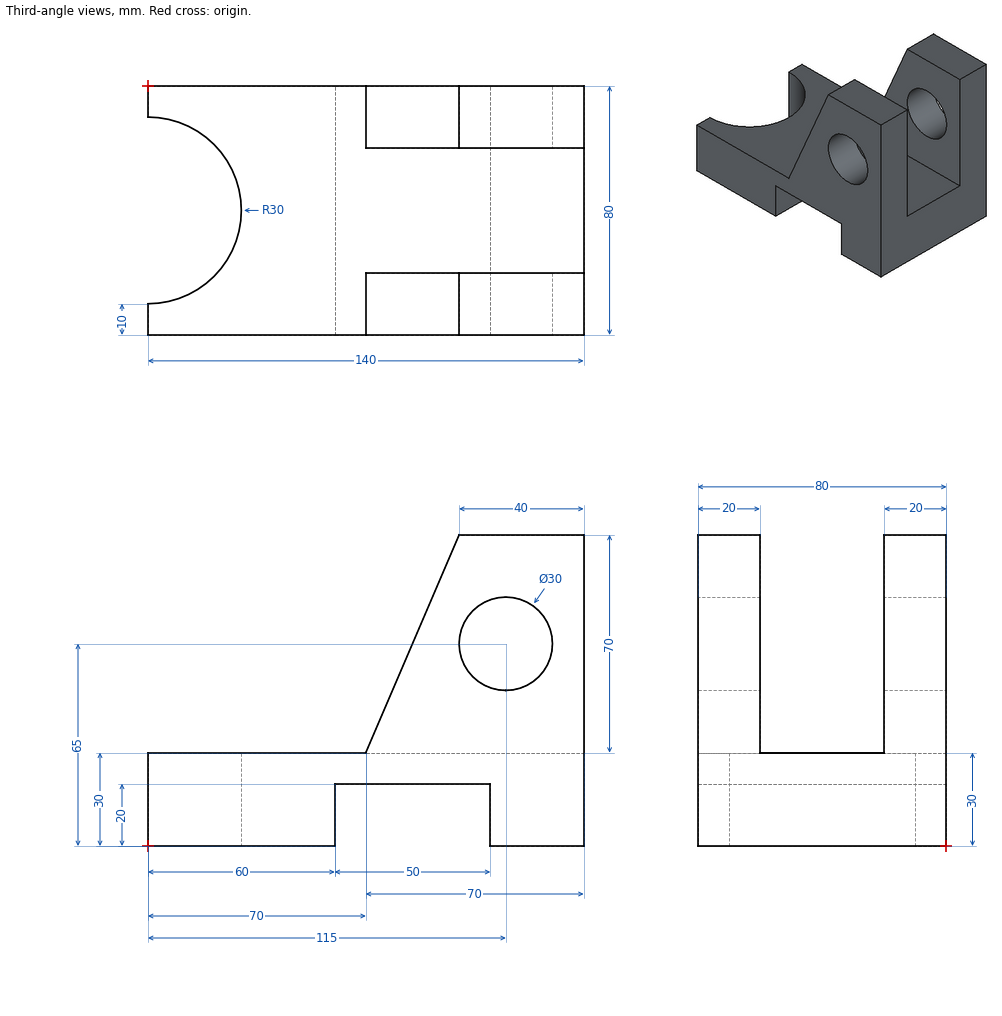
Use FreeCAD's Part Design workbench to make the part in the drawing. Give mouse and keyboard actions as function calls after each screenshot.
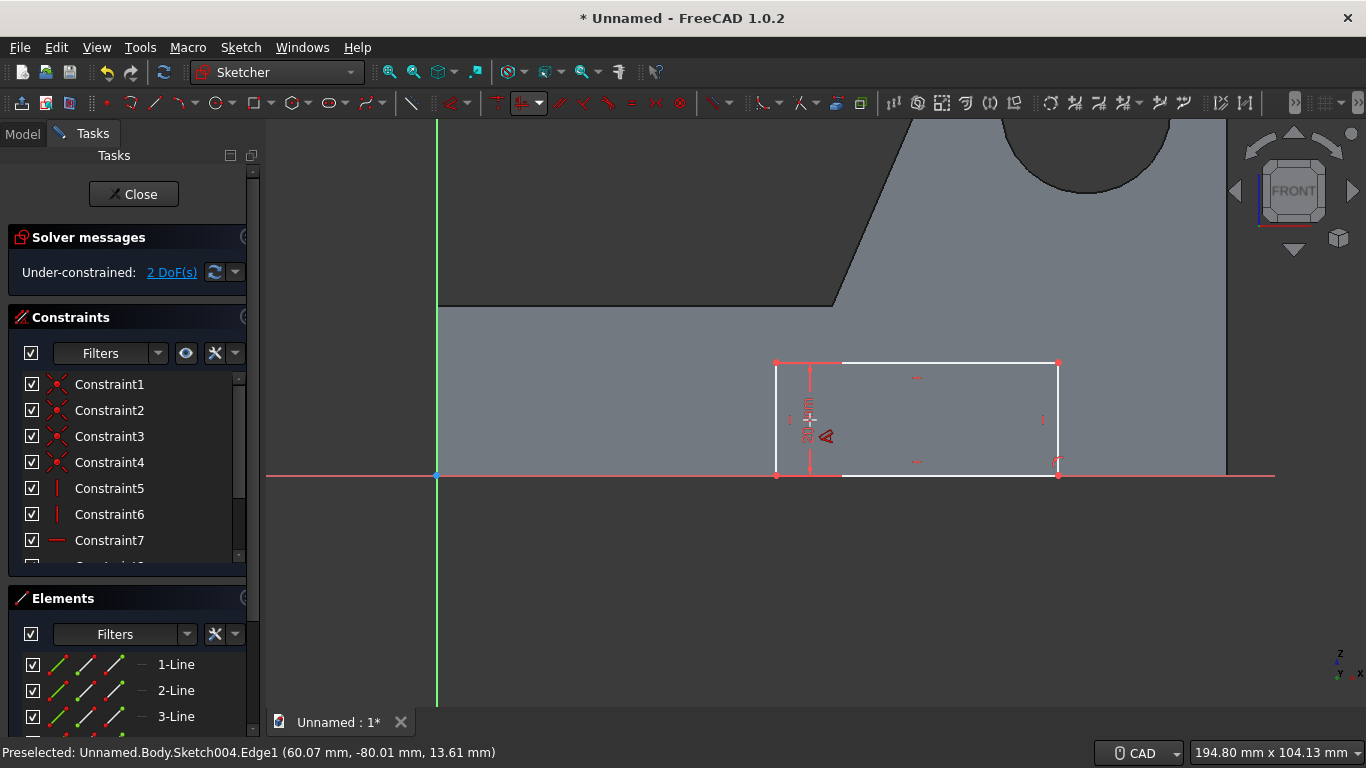
click(861, 476)
click(917, 510)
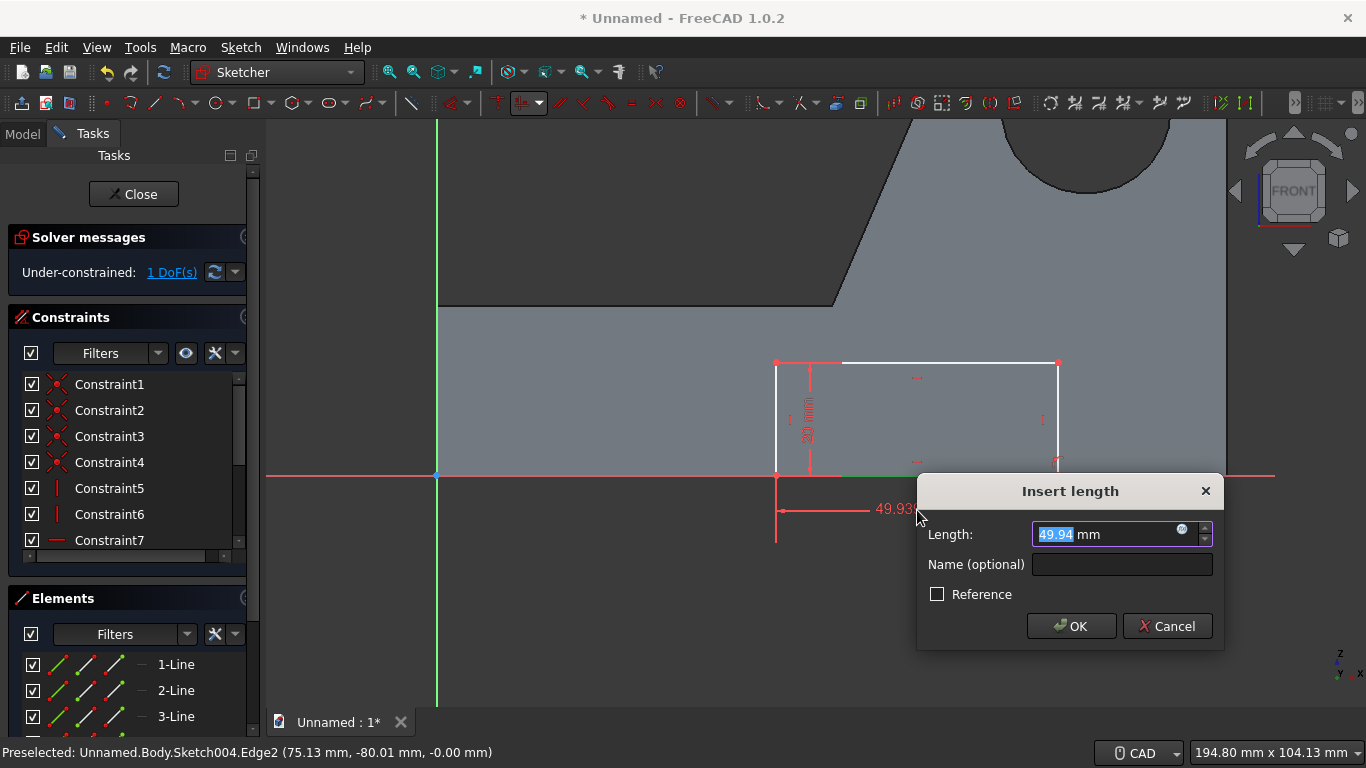
text(50)
key(Return)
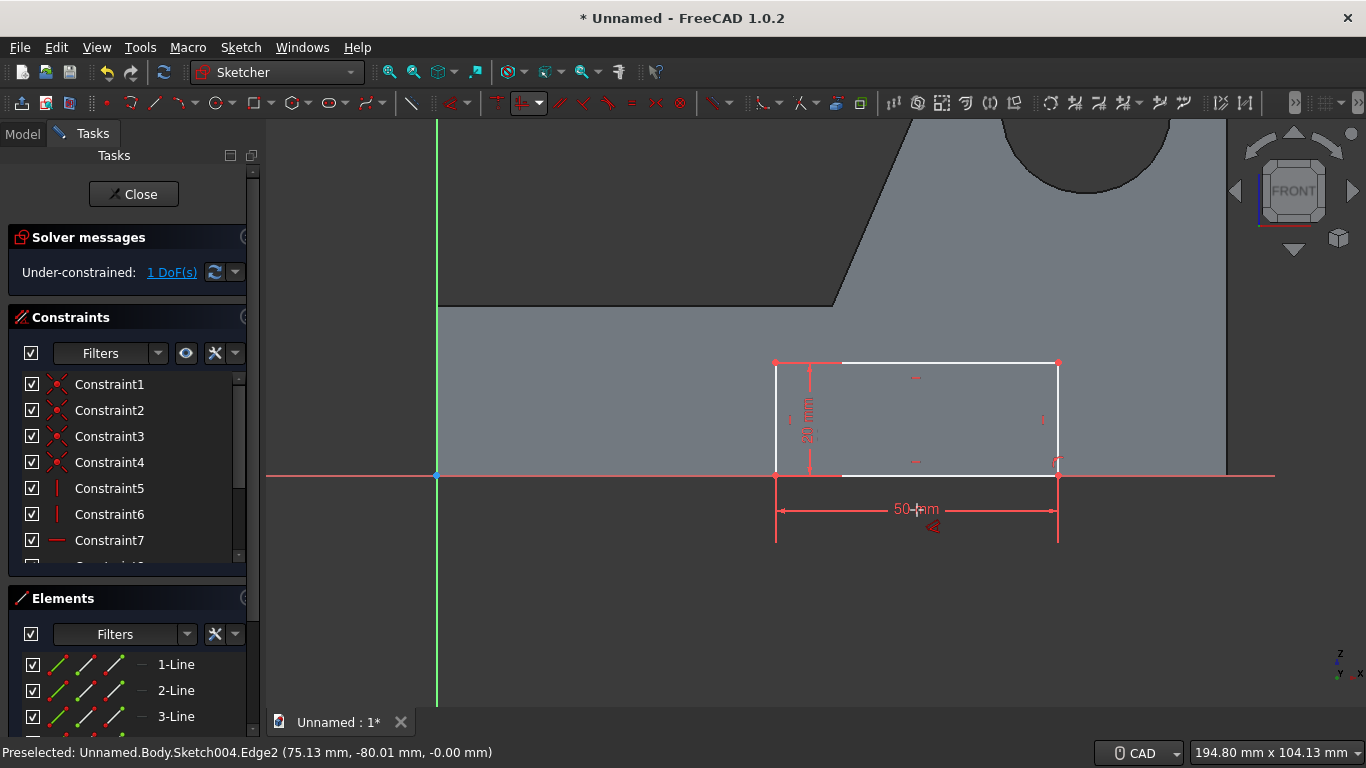
click(776, 363)
click(606, 510)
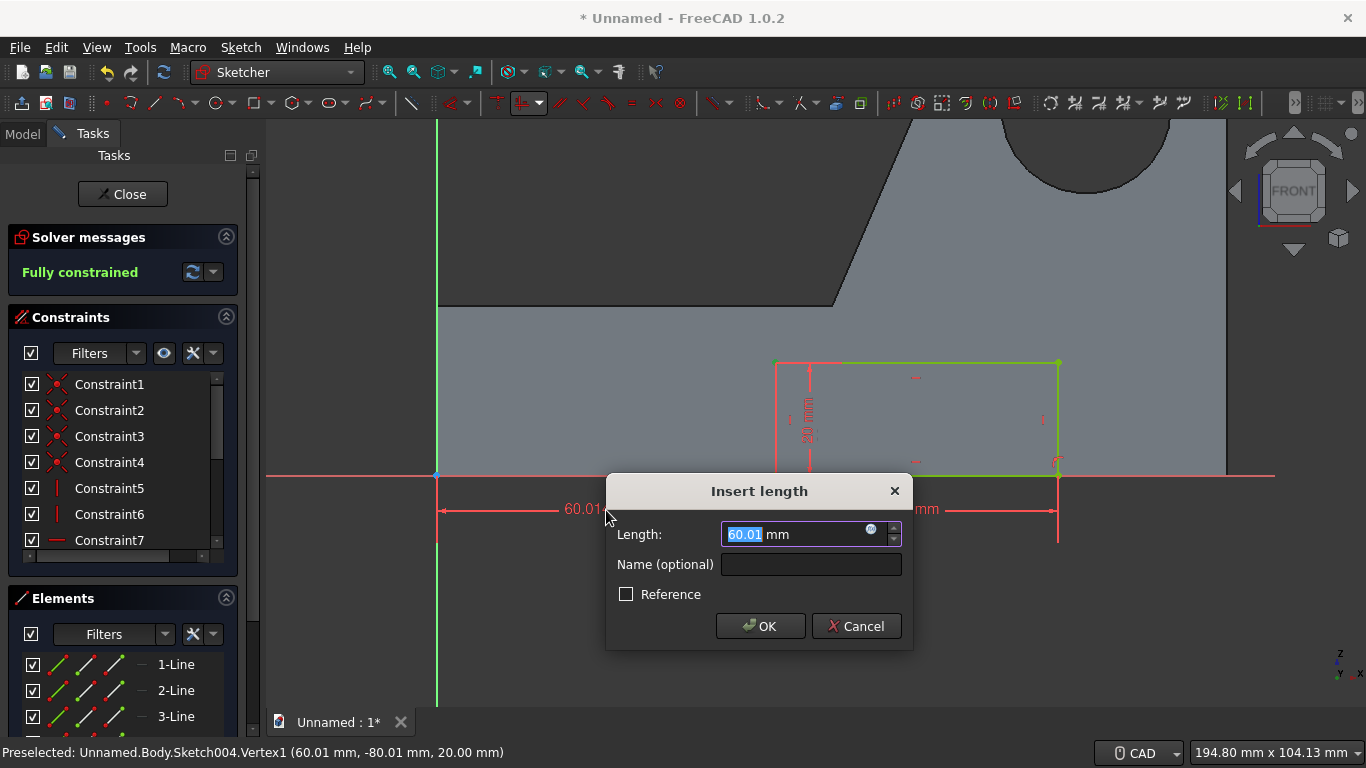
text(60)
key(Return)
key(Escape)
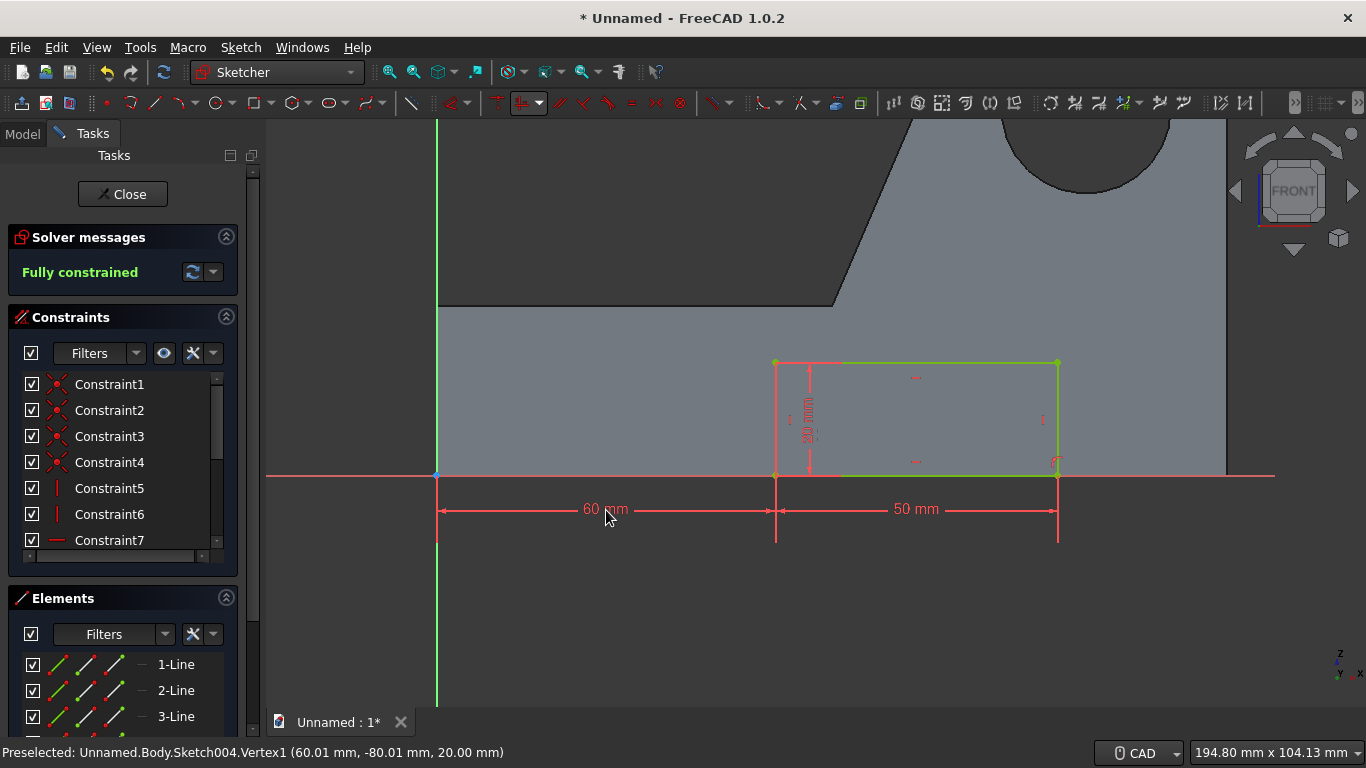
click(123, 194)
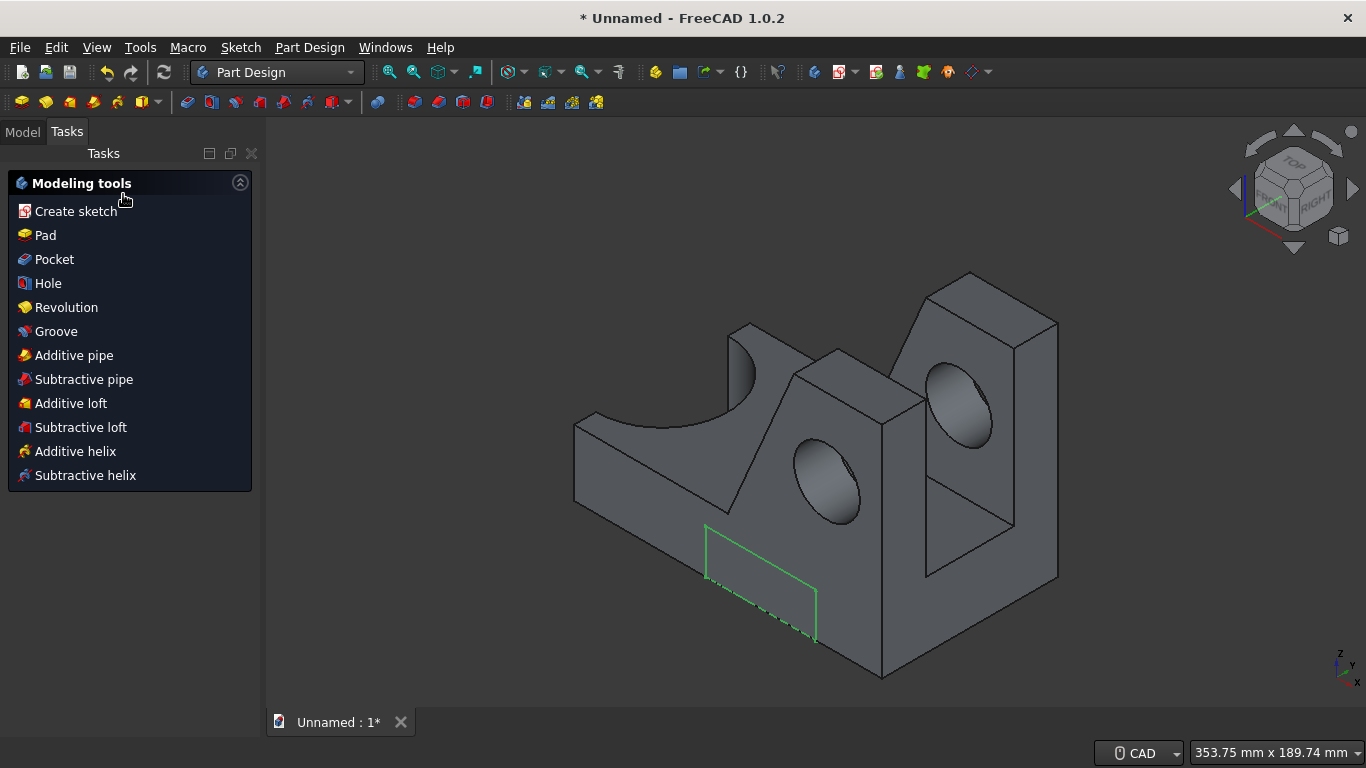
click(188, 102)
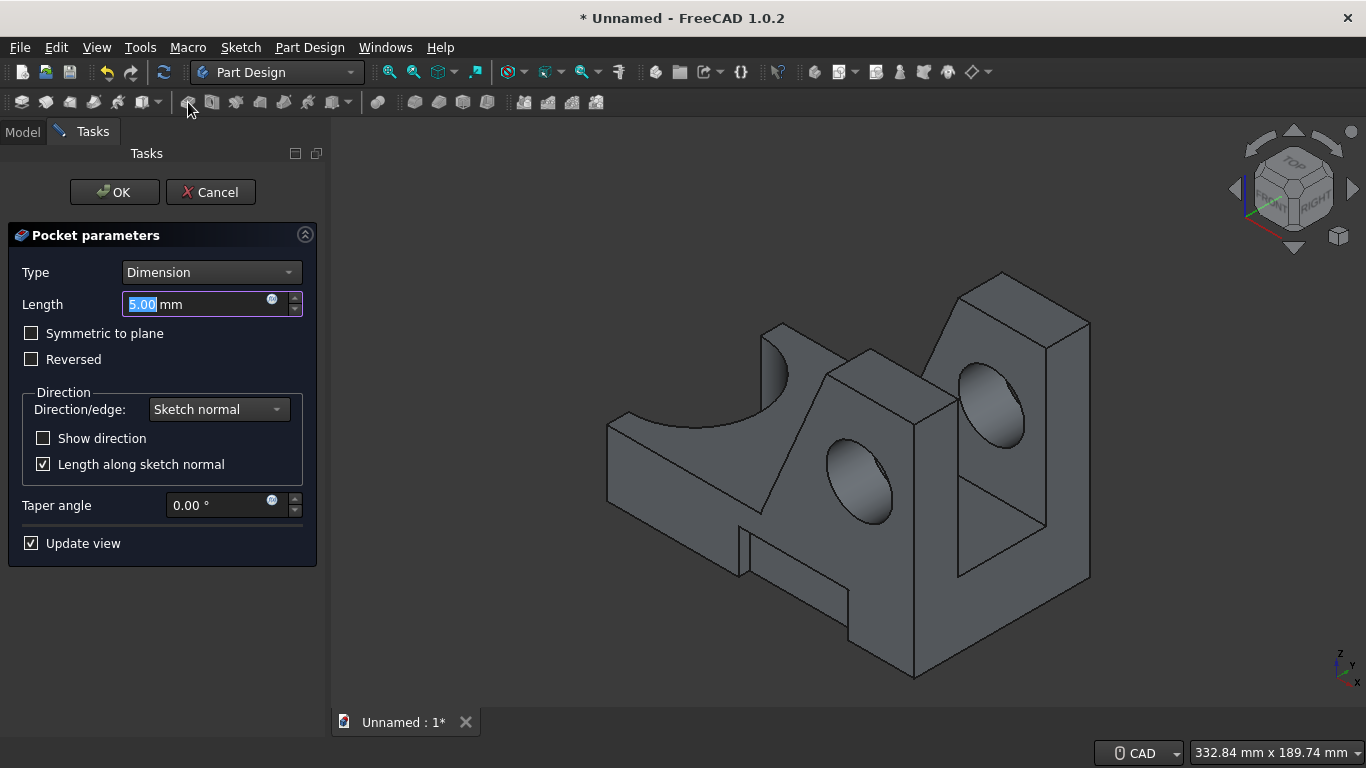
text(80)
key(Tab)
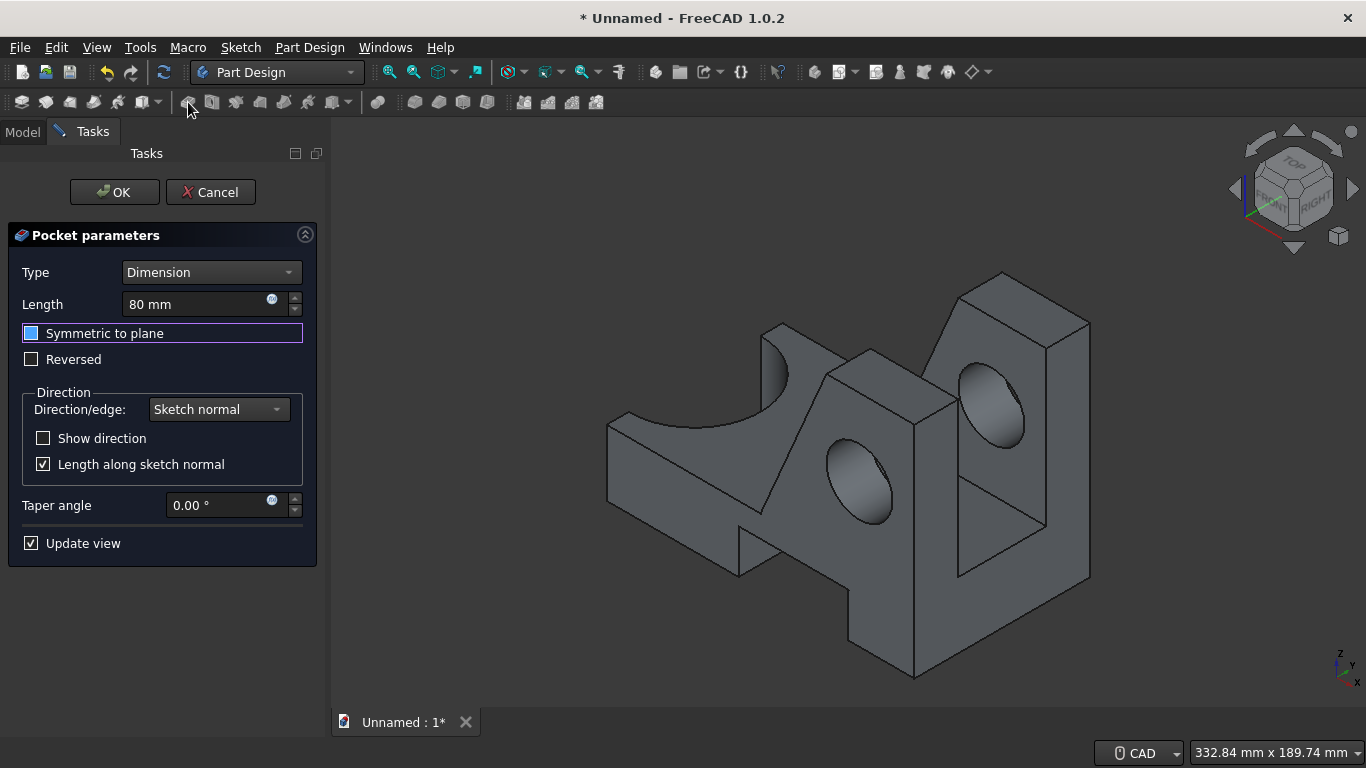
click(115, 192)